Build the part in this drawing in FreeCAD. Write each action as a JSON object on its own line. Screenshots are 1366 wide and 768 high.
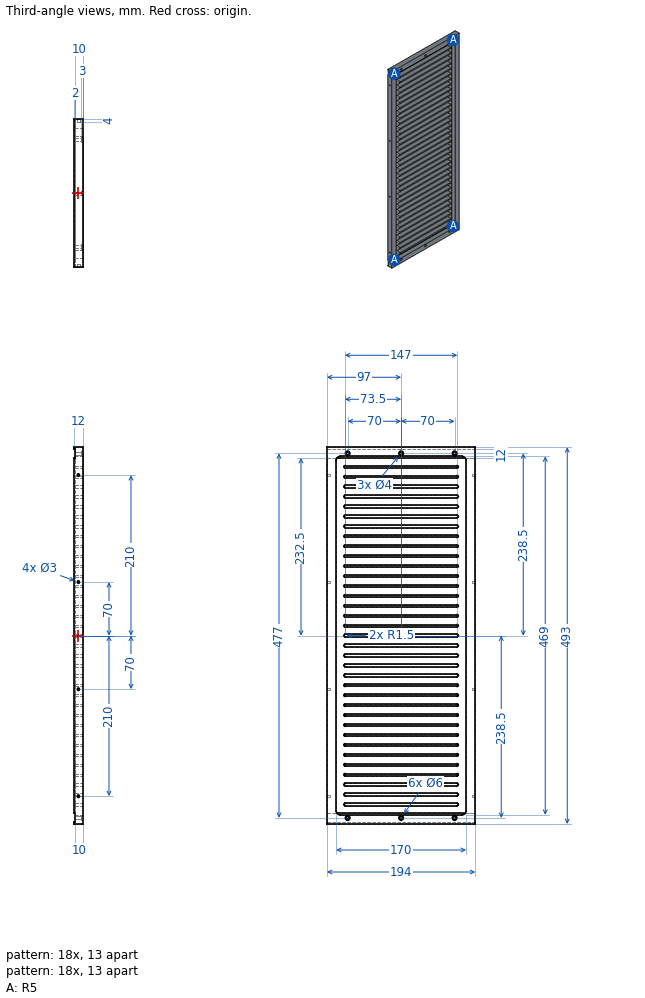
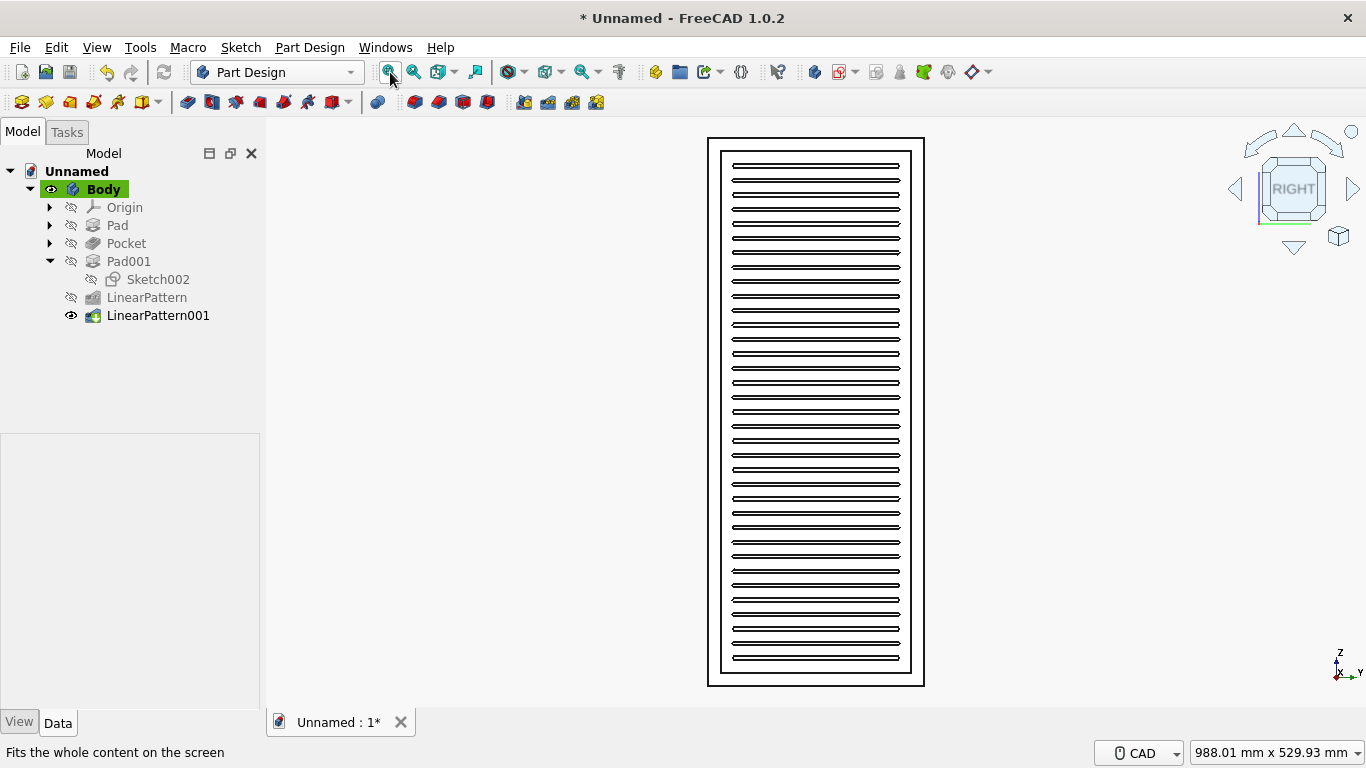
{"action": "scroll", "coordinate": [721, 672], "scroll_direction": "up", "scroll_amount": 7}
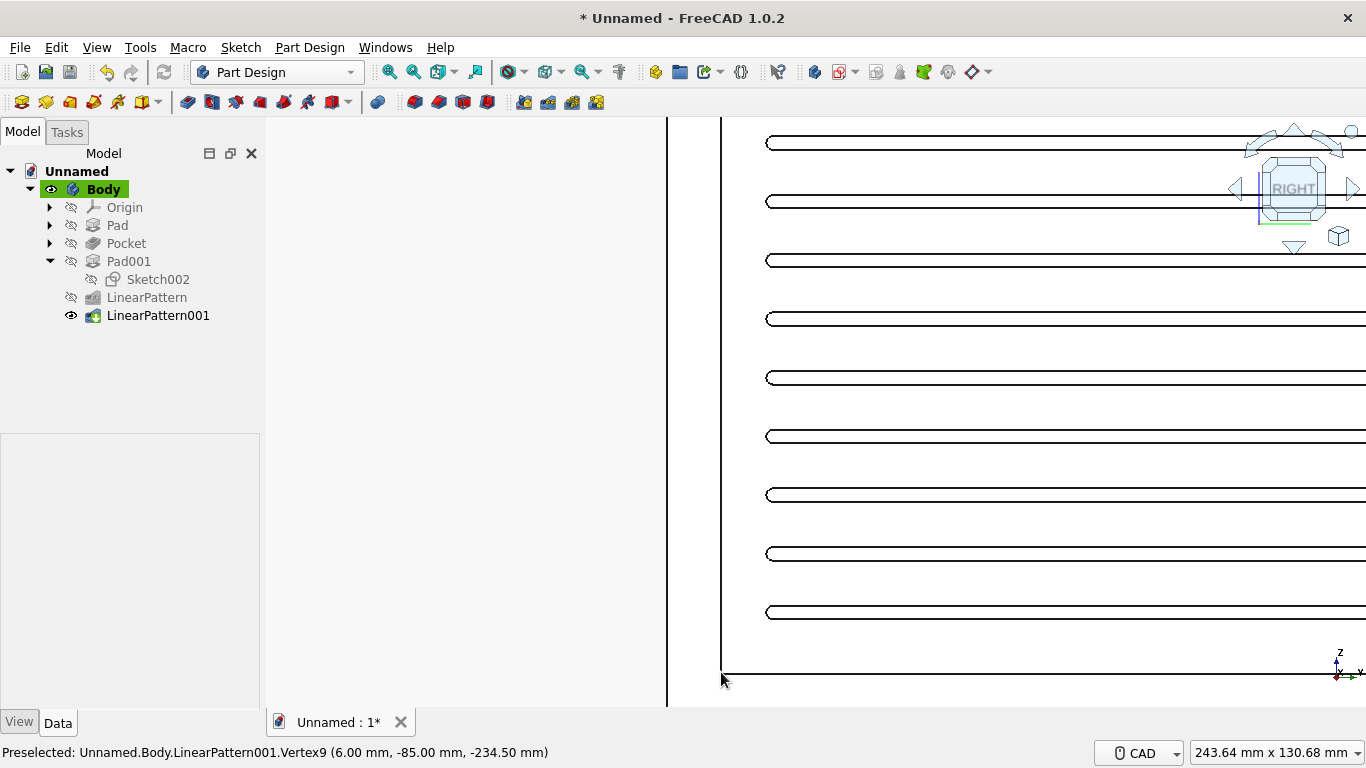
{"action": "left_click", "coordinate": [390, 72]}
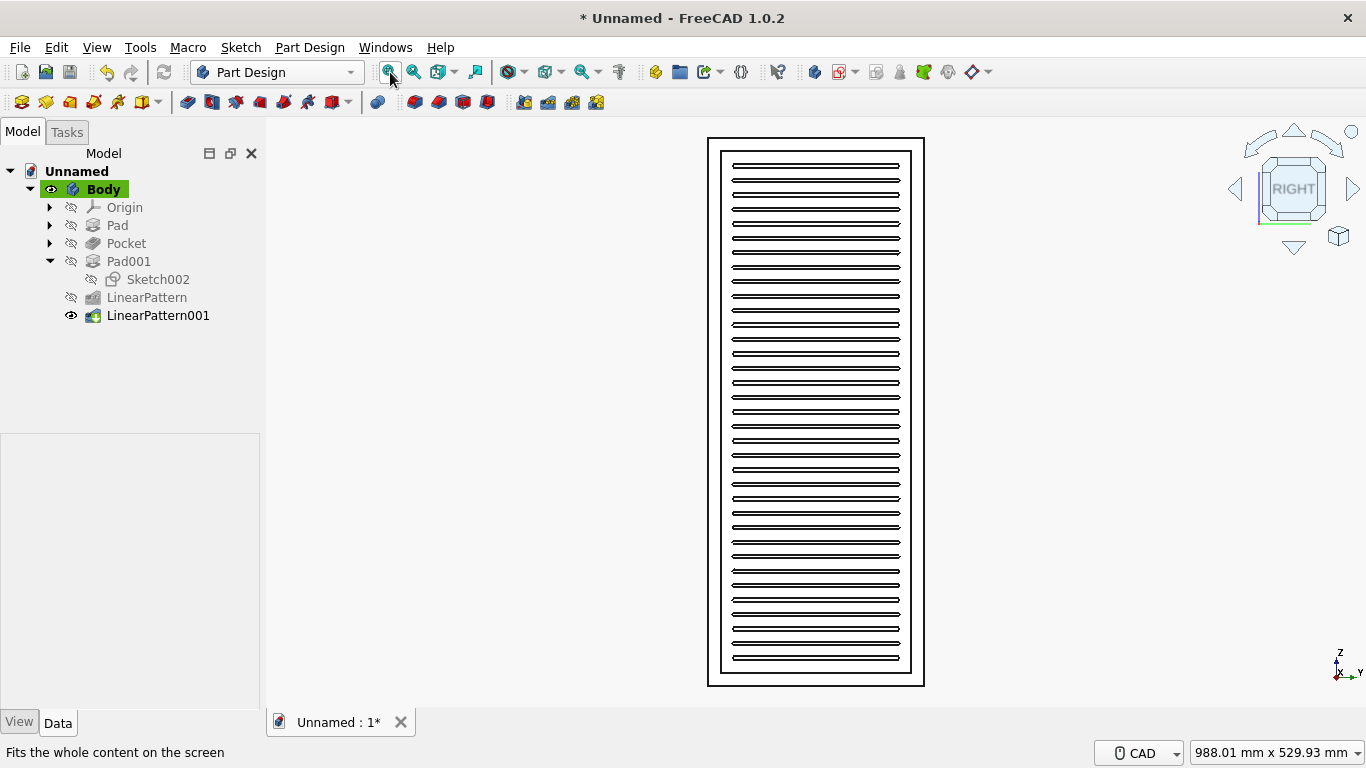
{"action": "key", "text": "5"}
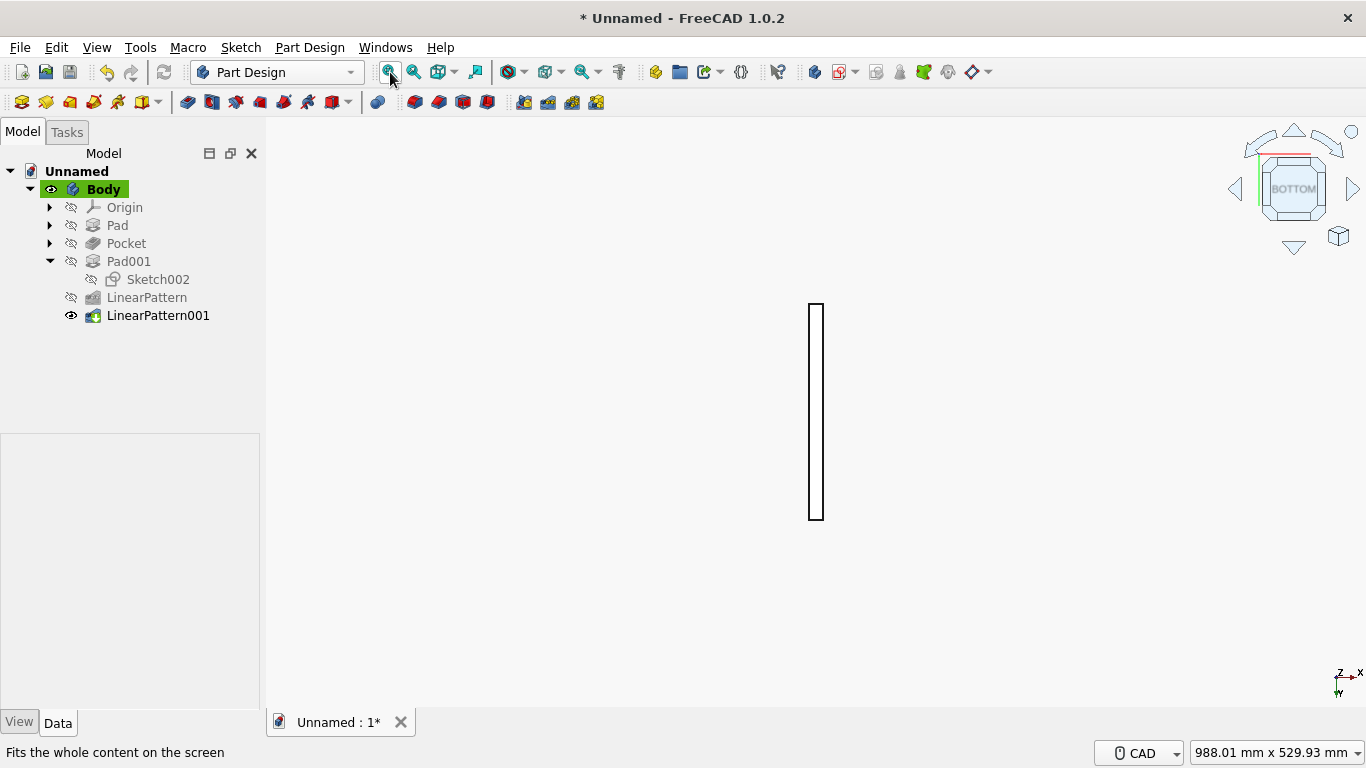
{"action": "left_click", "coordinate": [390, 72]}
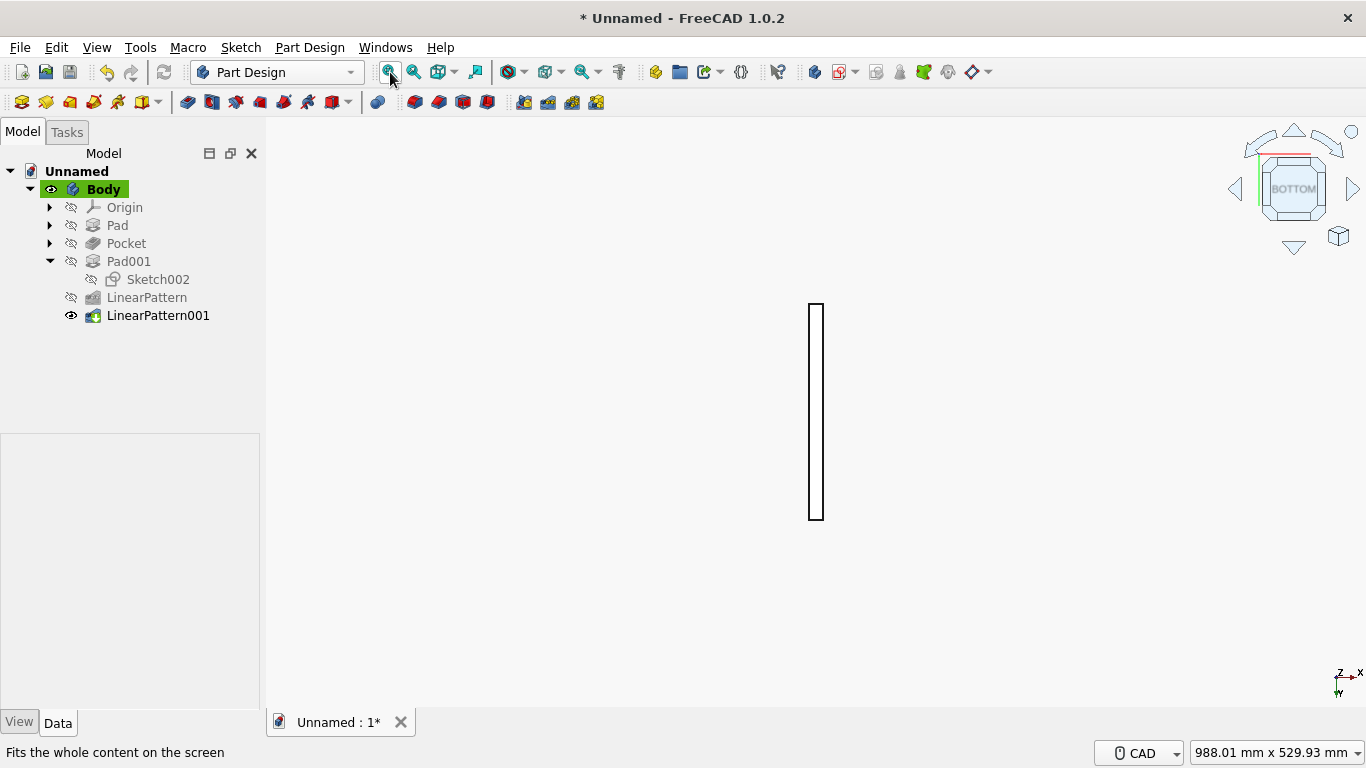
{"action": "scroll", "coordinate": [817, 316], "scroll_direction": "up", "scroll_amount": 7}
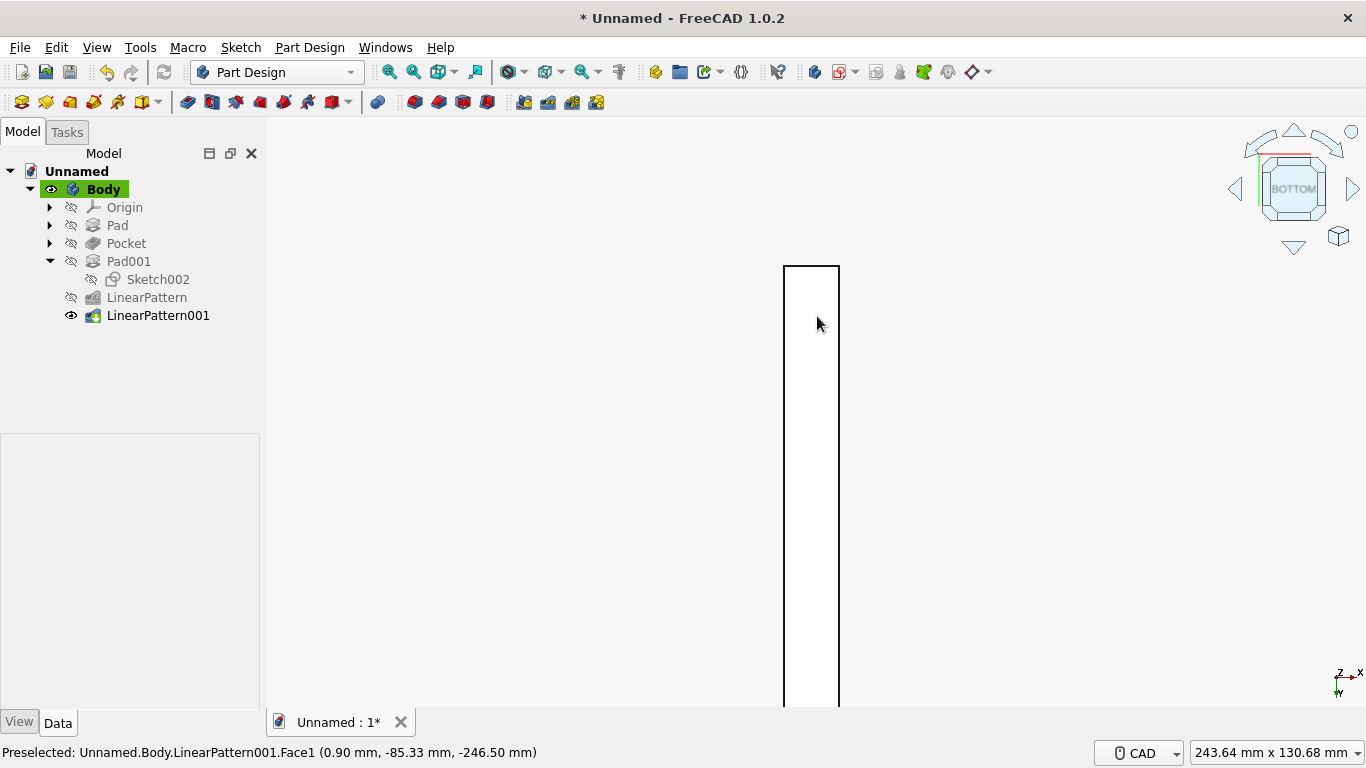
{"action": "key", "text": "v f"}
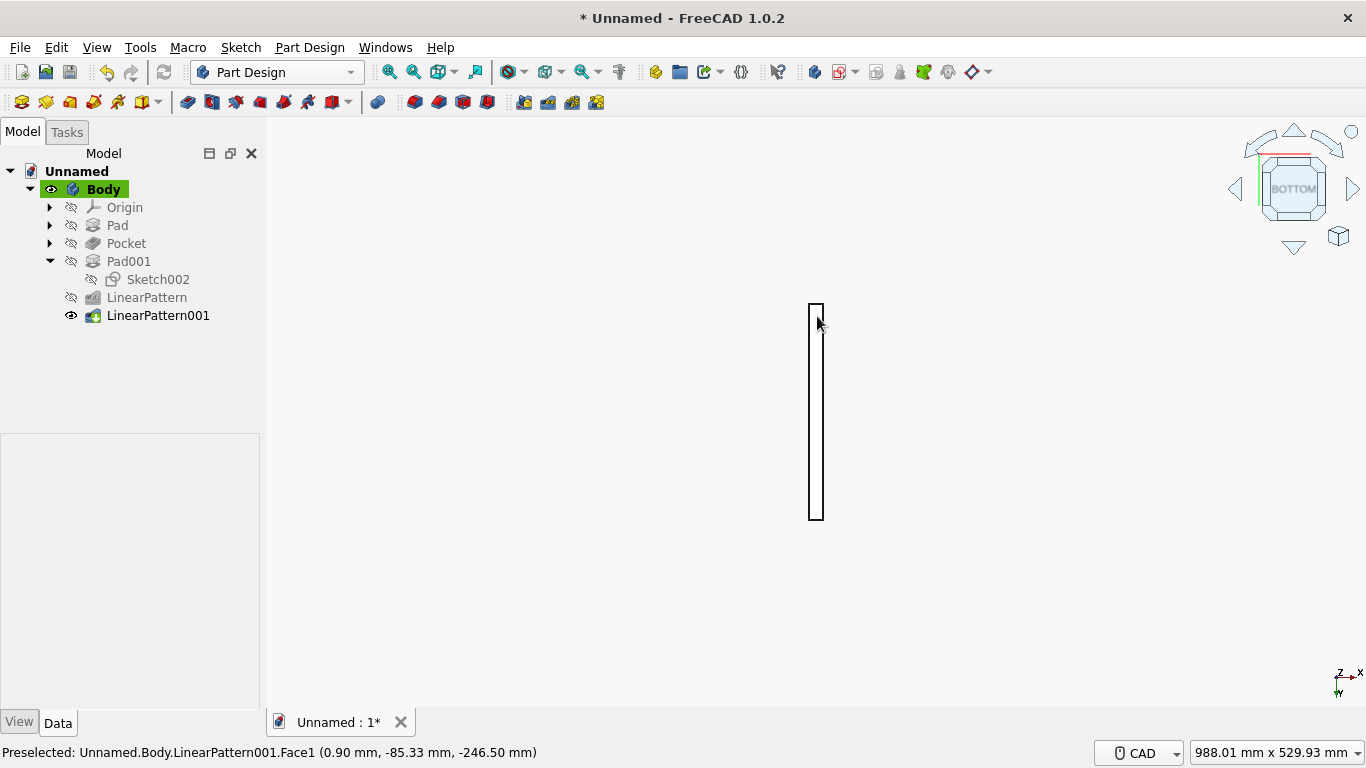
{"action": "key", "text": "4"}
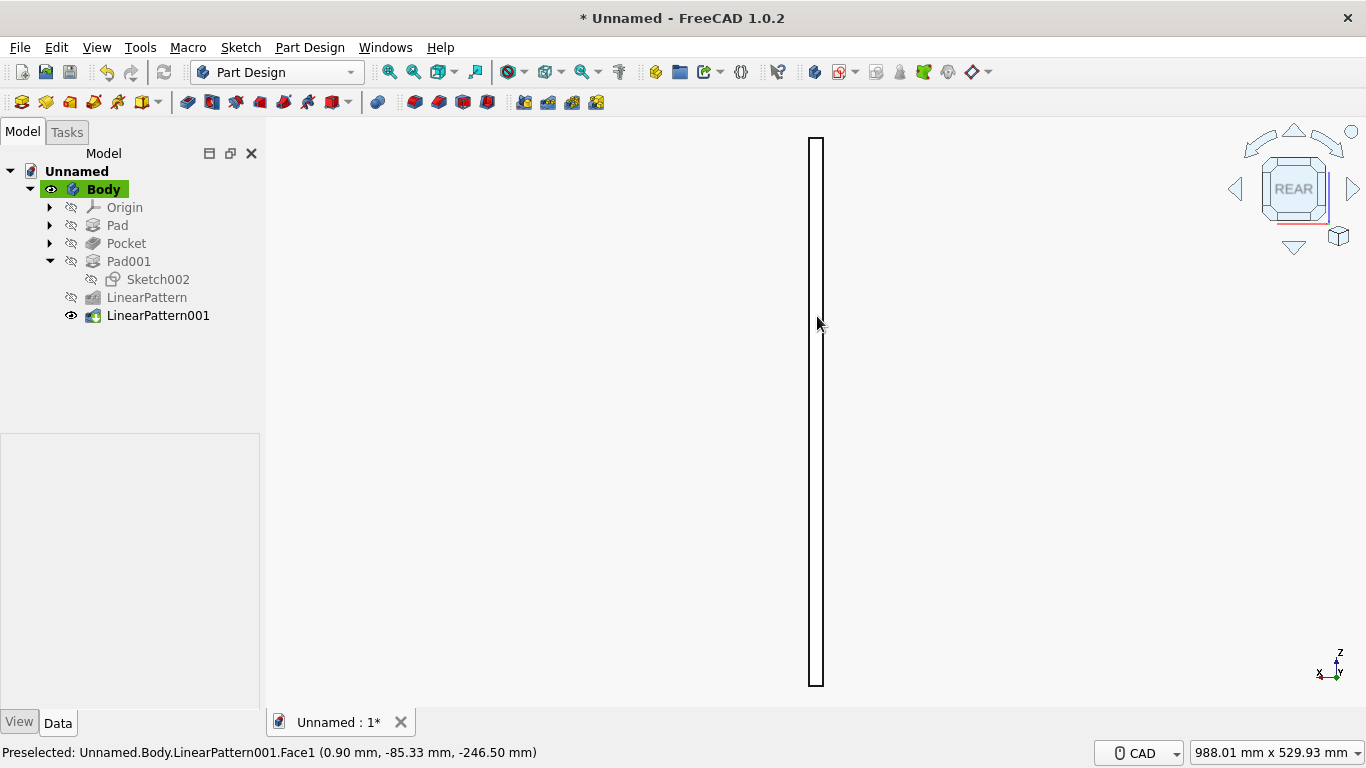
{"action": "scroll", "coordinate": [815, 672], "scroll_direction": "up", "scroll_amount": 7}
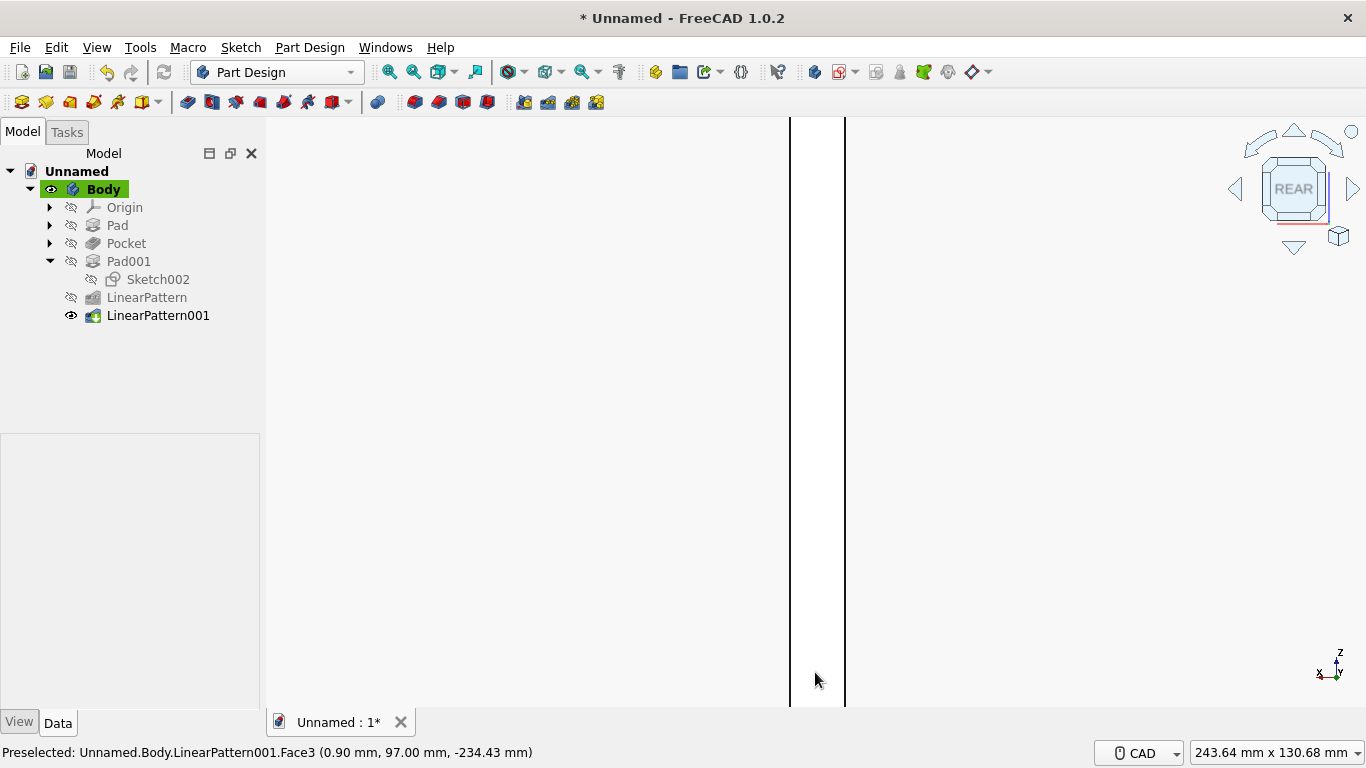
{"action": "key", "text": "v f"}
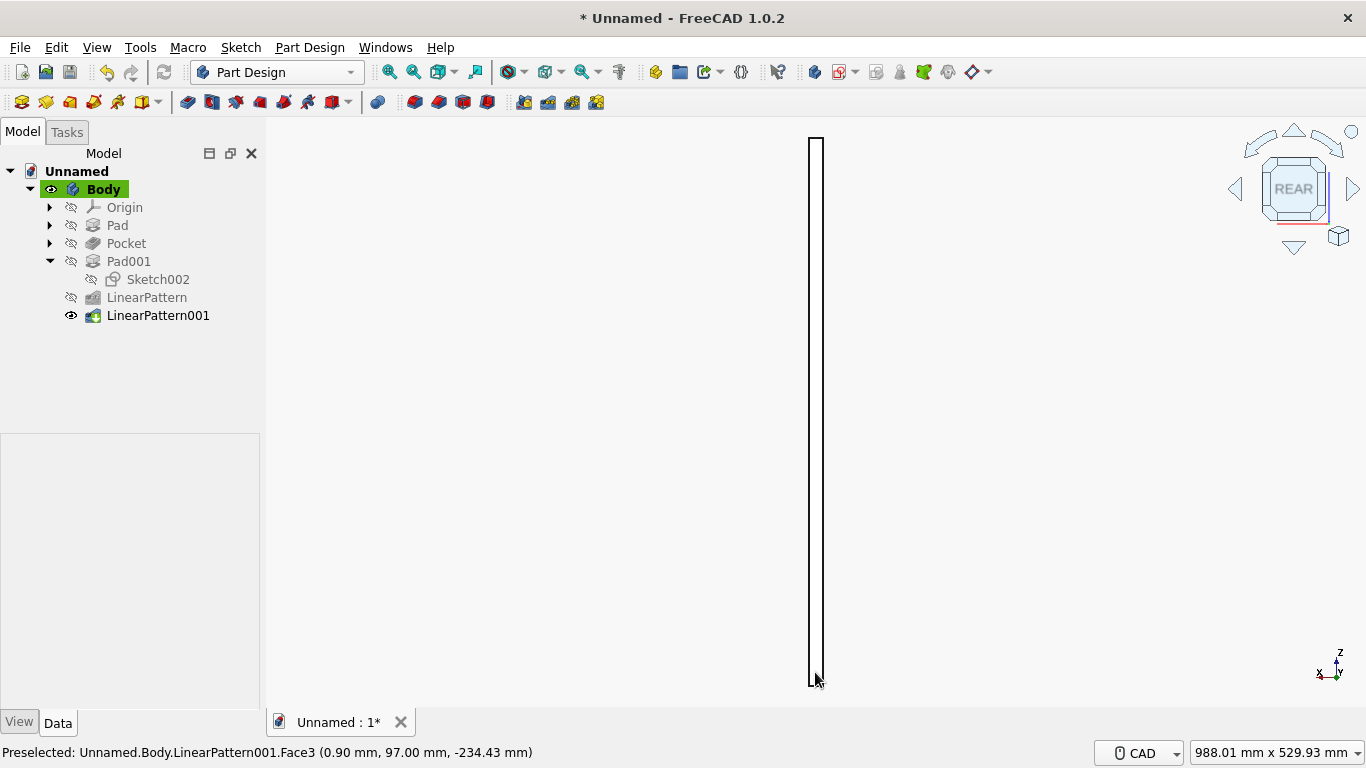
{"action": "key", "text": "6"}